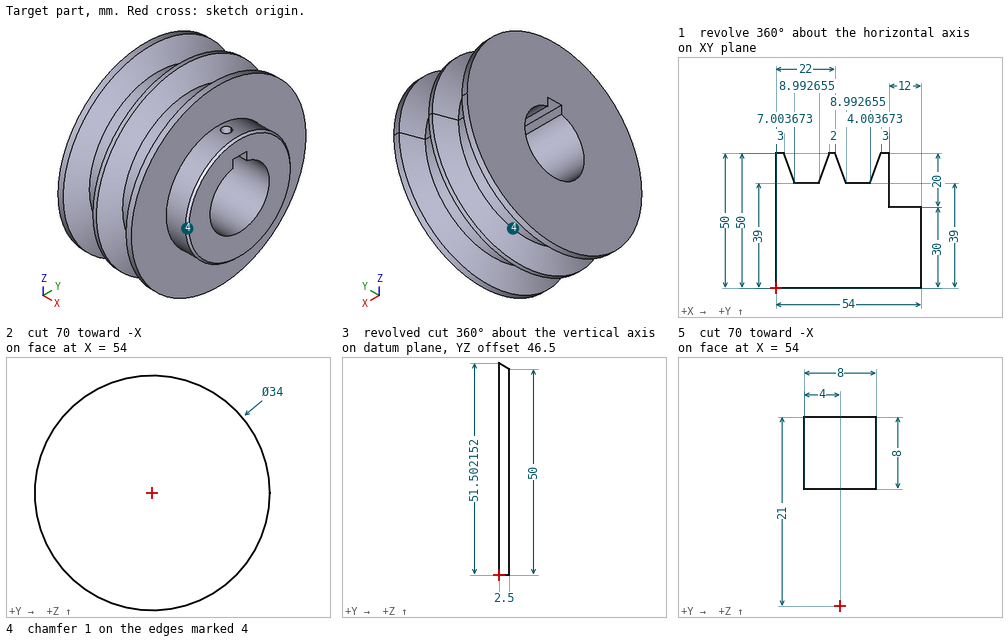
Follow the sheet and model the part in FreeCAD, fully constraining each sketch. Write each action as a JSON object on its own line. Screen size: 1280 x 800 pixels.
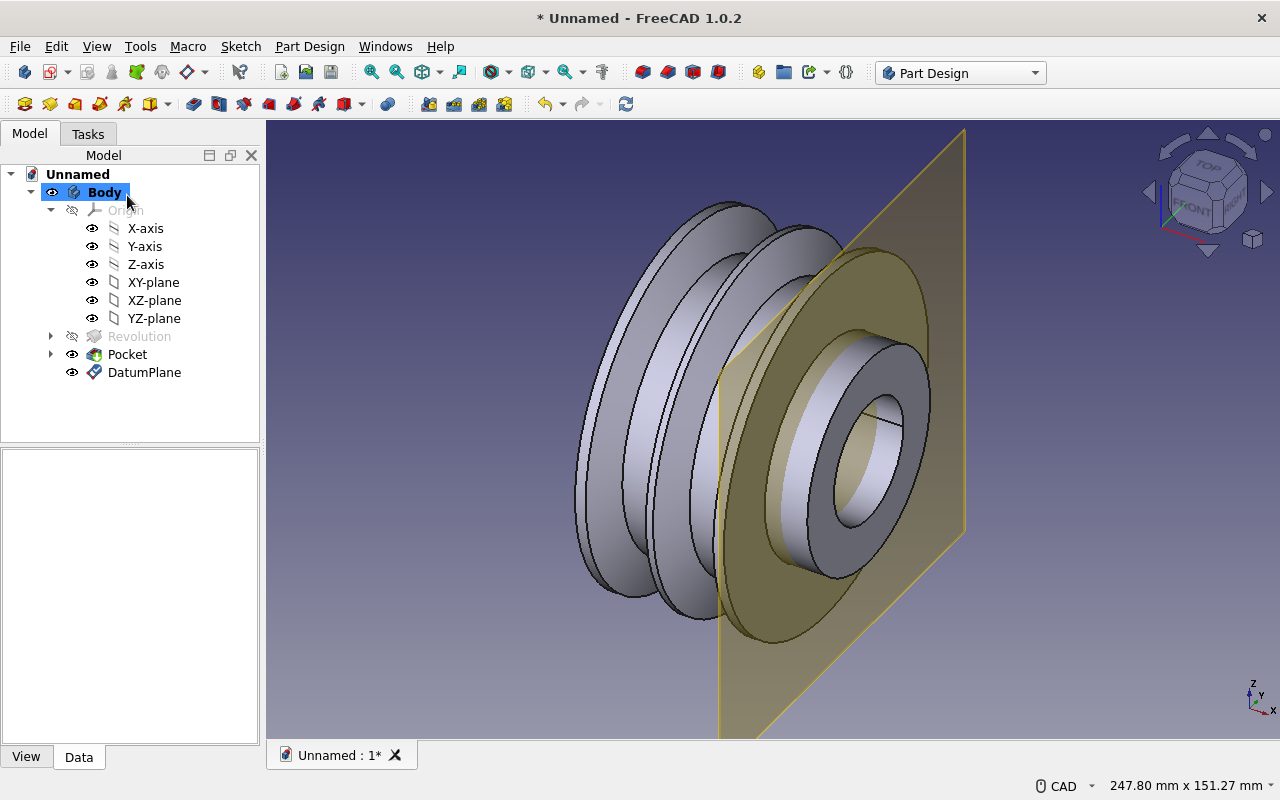
{"action": "left_click", "coordinate": [117, 372]}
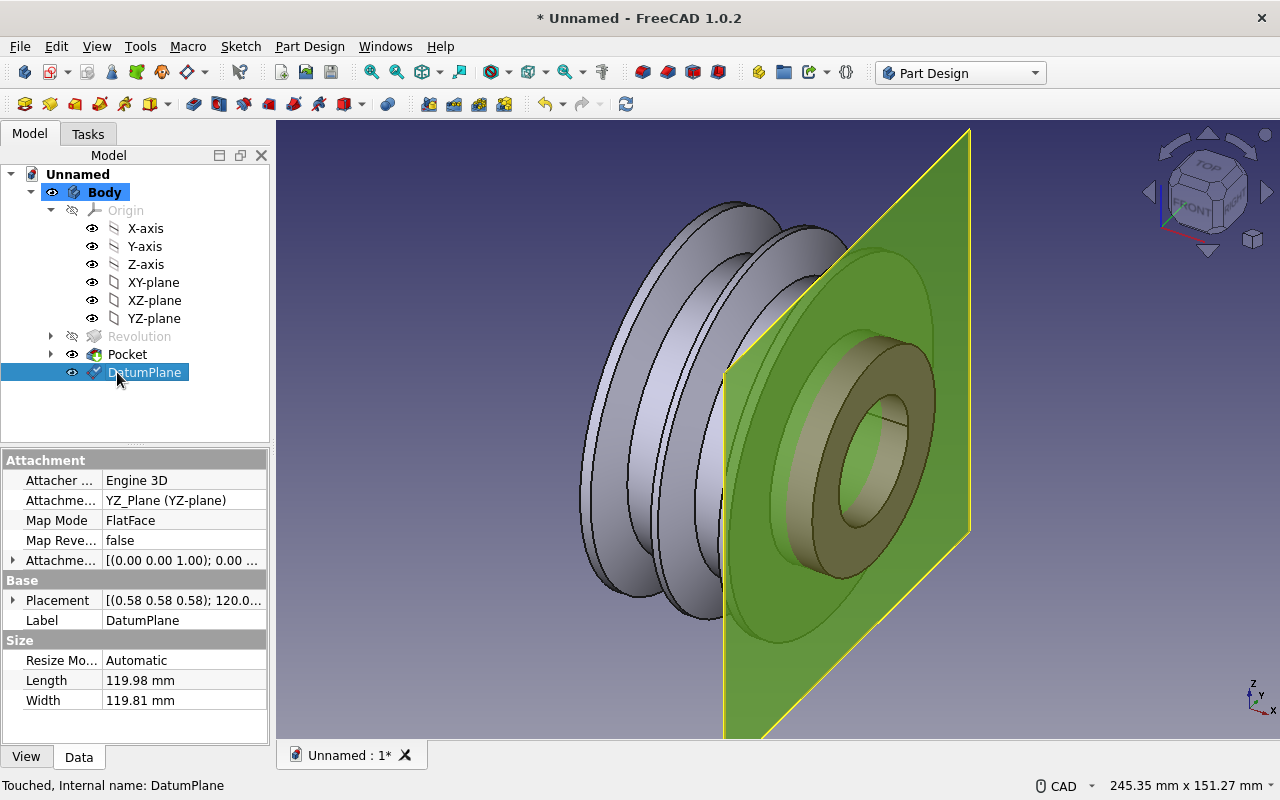
{"action": "left_click", "coordinate": [50, 72]}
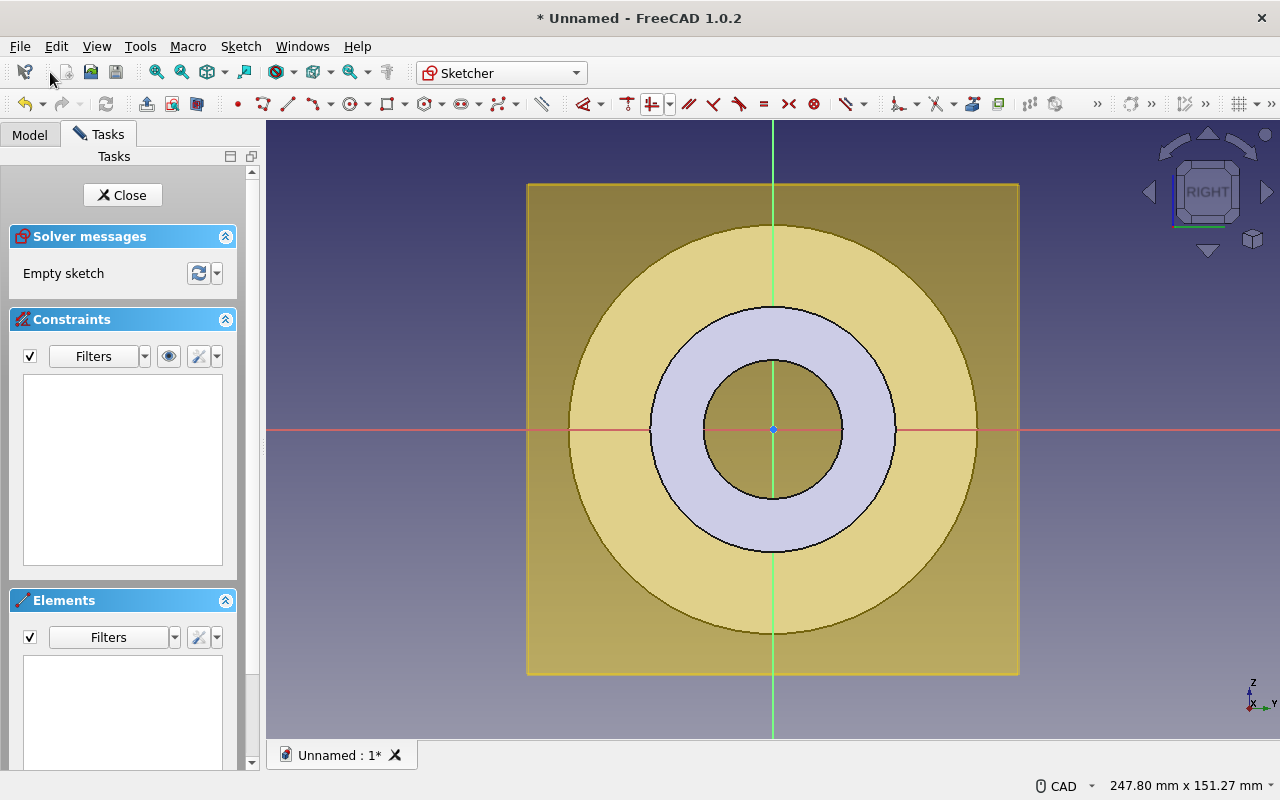
{"action": "key", "text": "q s"}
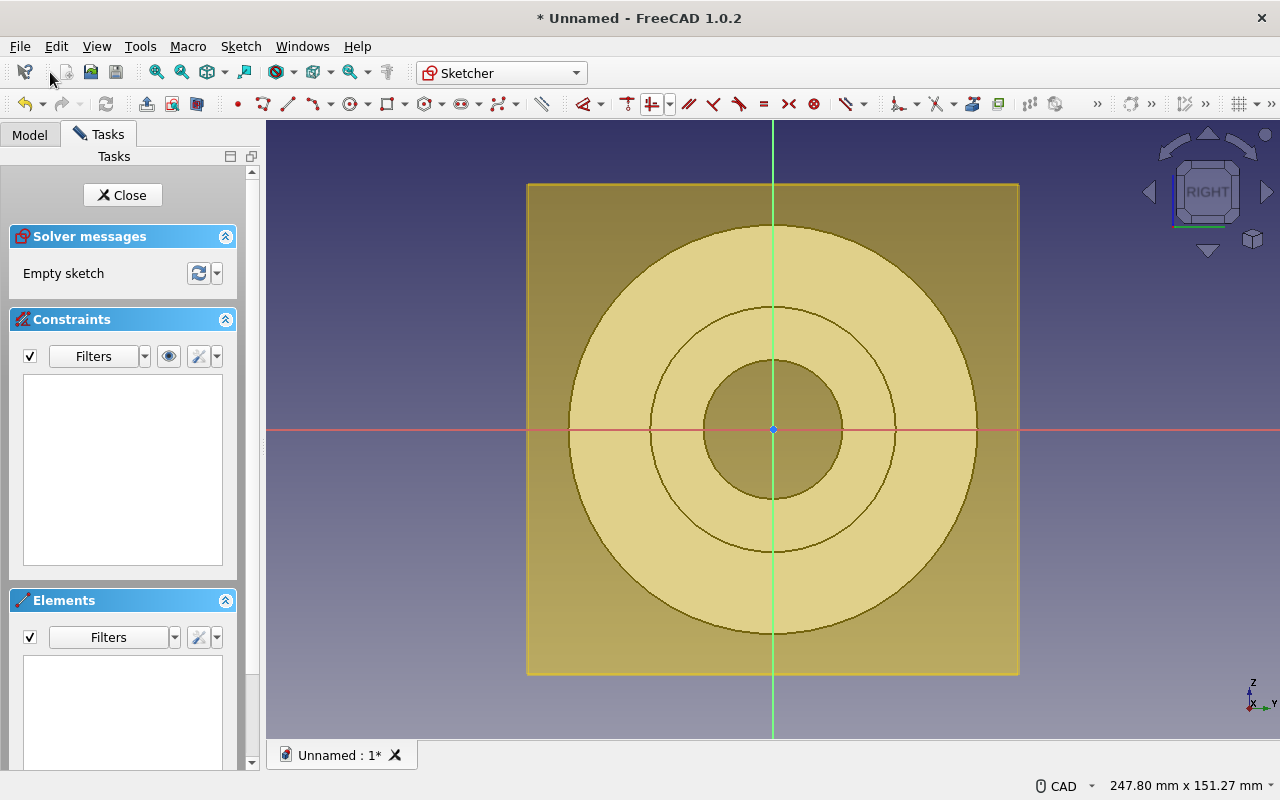
{"action": "scroll", "coordinate": [868, 196], "scroll_direction": "up", "scroll_amount": 3}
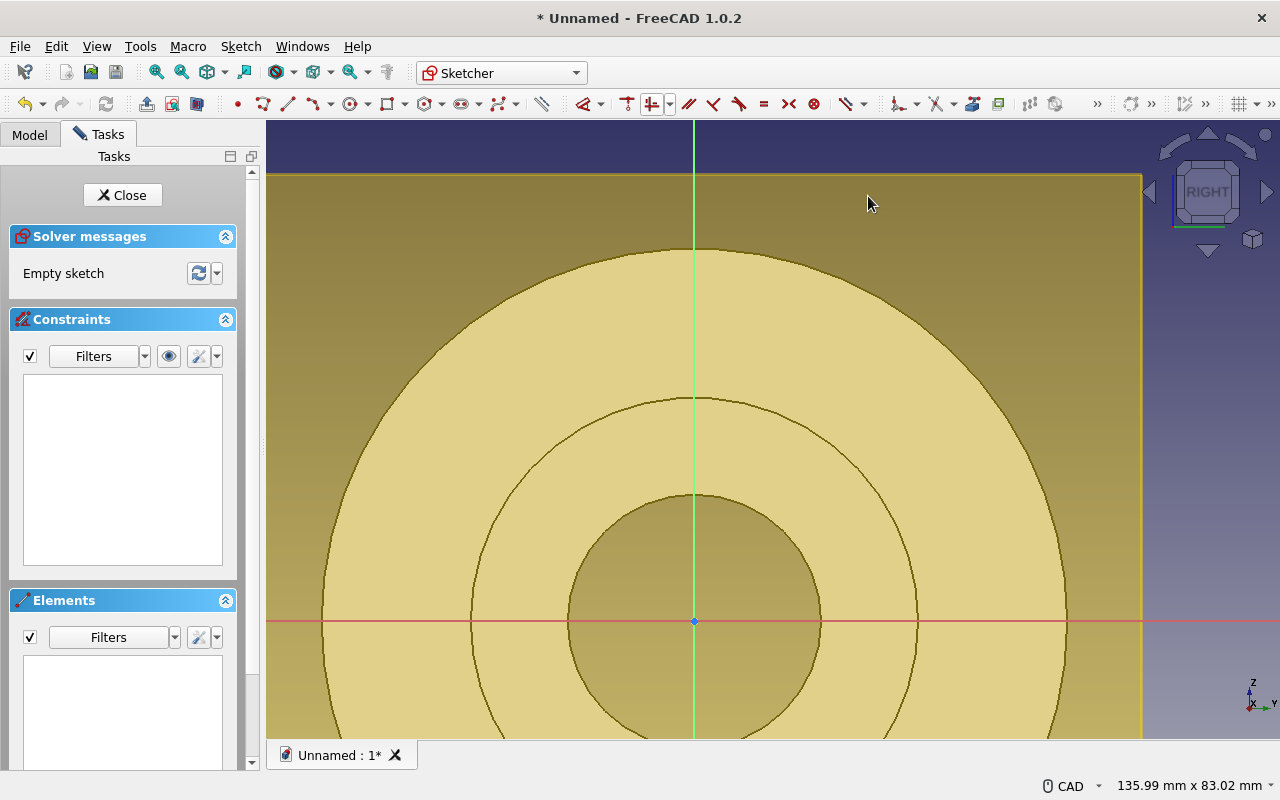
{"action": "key", "text": "g m"}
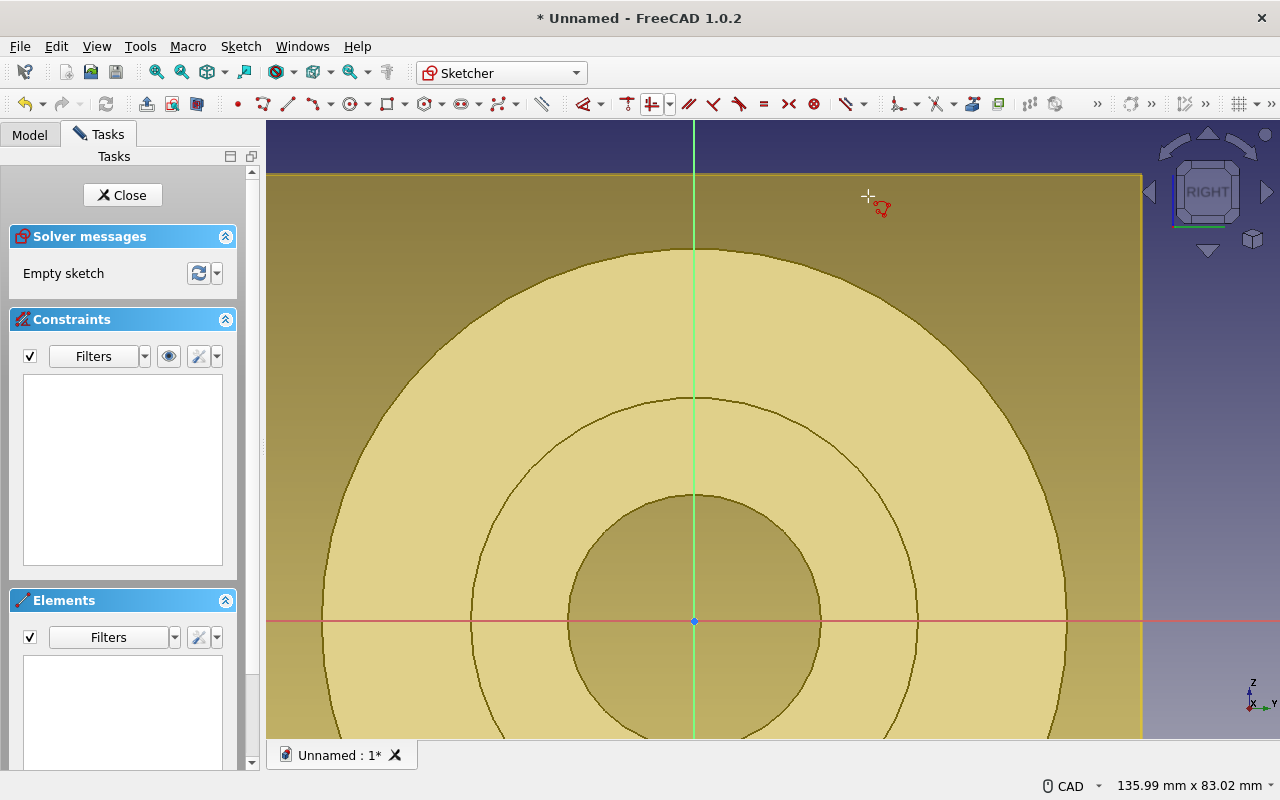
{"action": "left_click", "coordinate": [694, 621]}
{"action": "left_click", "coordinate": [713, 612]}
{"action": "left_click", "coordinate": [713, 249]}
{"action": "left_click", "coordinate": [703, 237]}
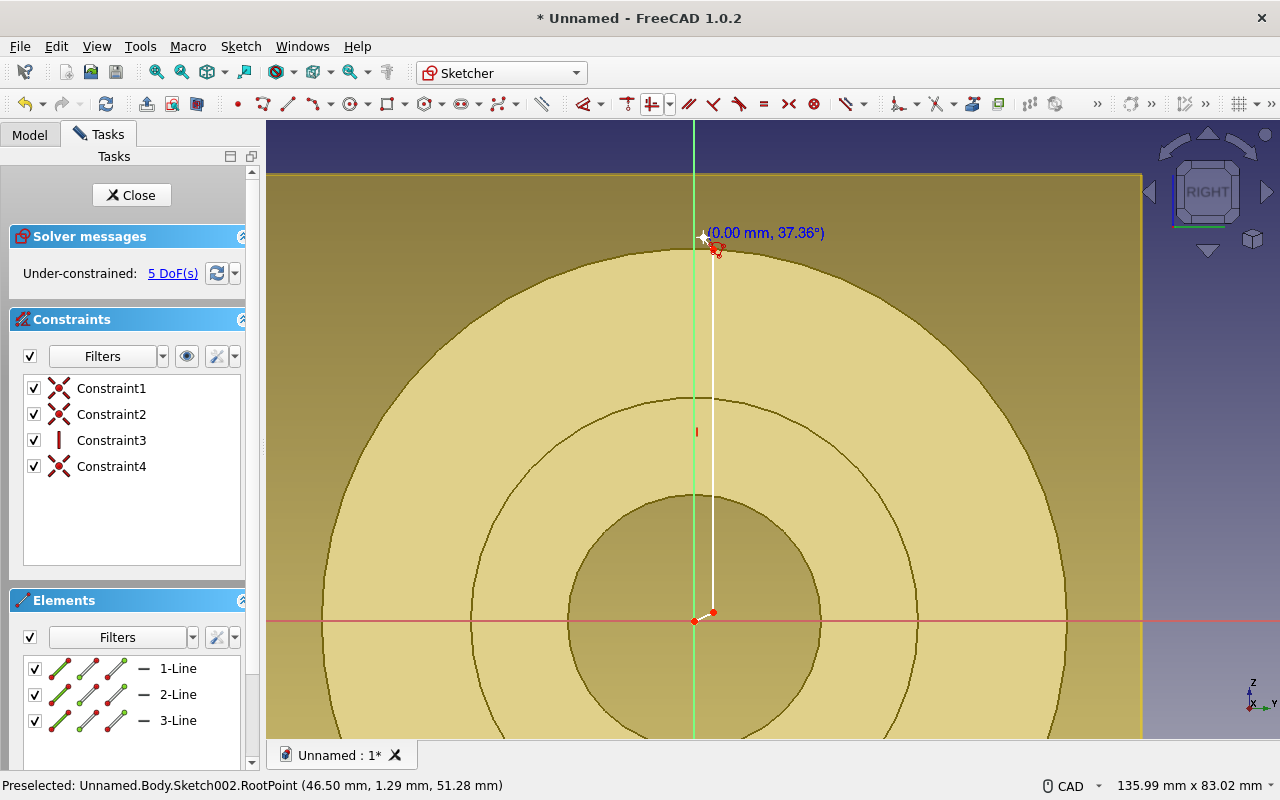
{"action": "scroll", "coordinate": [694, 621], "scroll_direction": "up", "scroll_amount": 3}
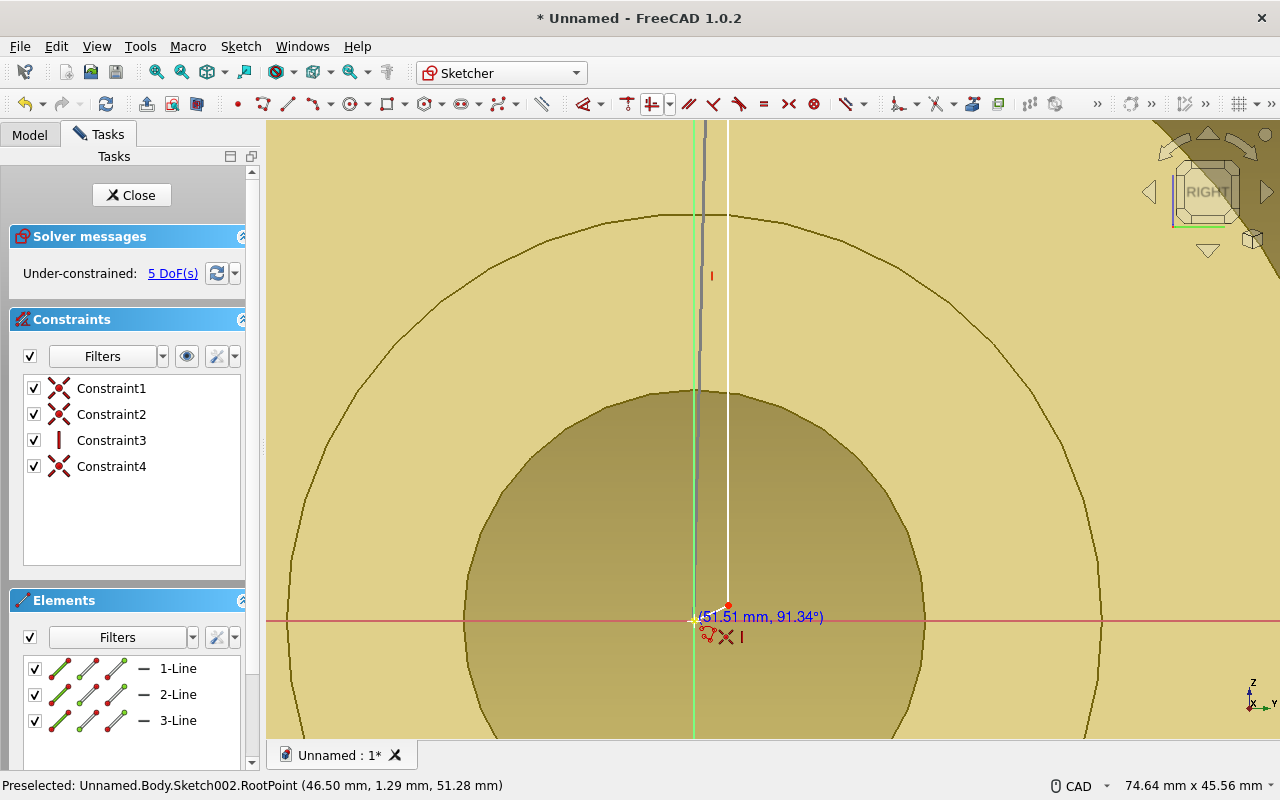
{"action": "left_click", "coordinate": [694, 621]}
{"action": "key", "text": "Escape"}
{"action": "key", "text": "Escape"}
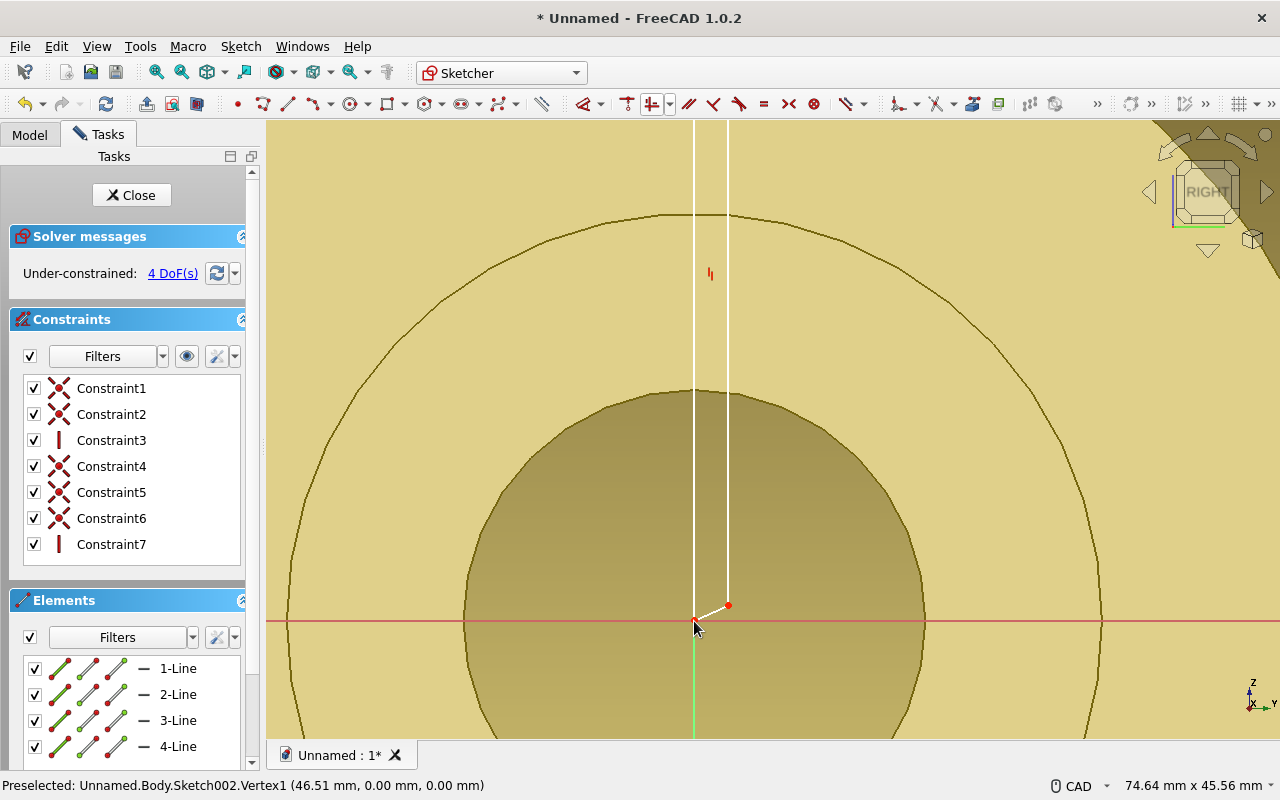
{"action": "scroll", "coordinate": [718, 610], "scroll_direction": "up", "scroll_amount": 2}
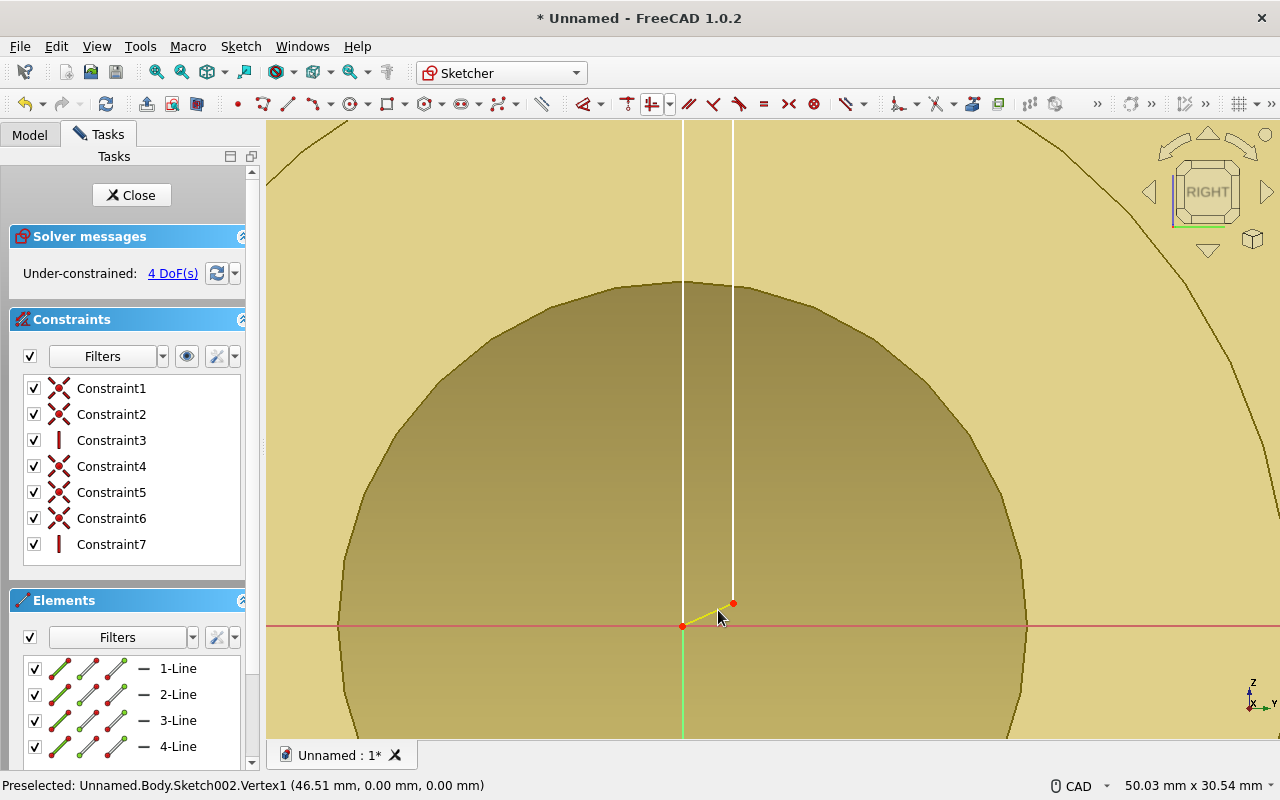
{"action": "left_click", "coordinate": [718, 610]}